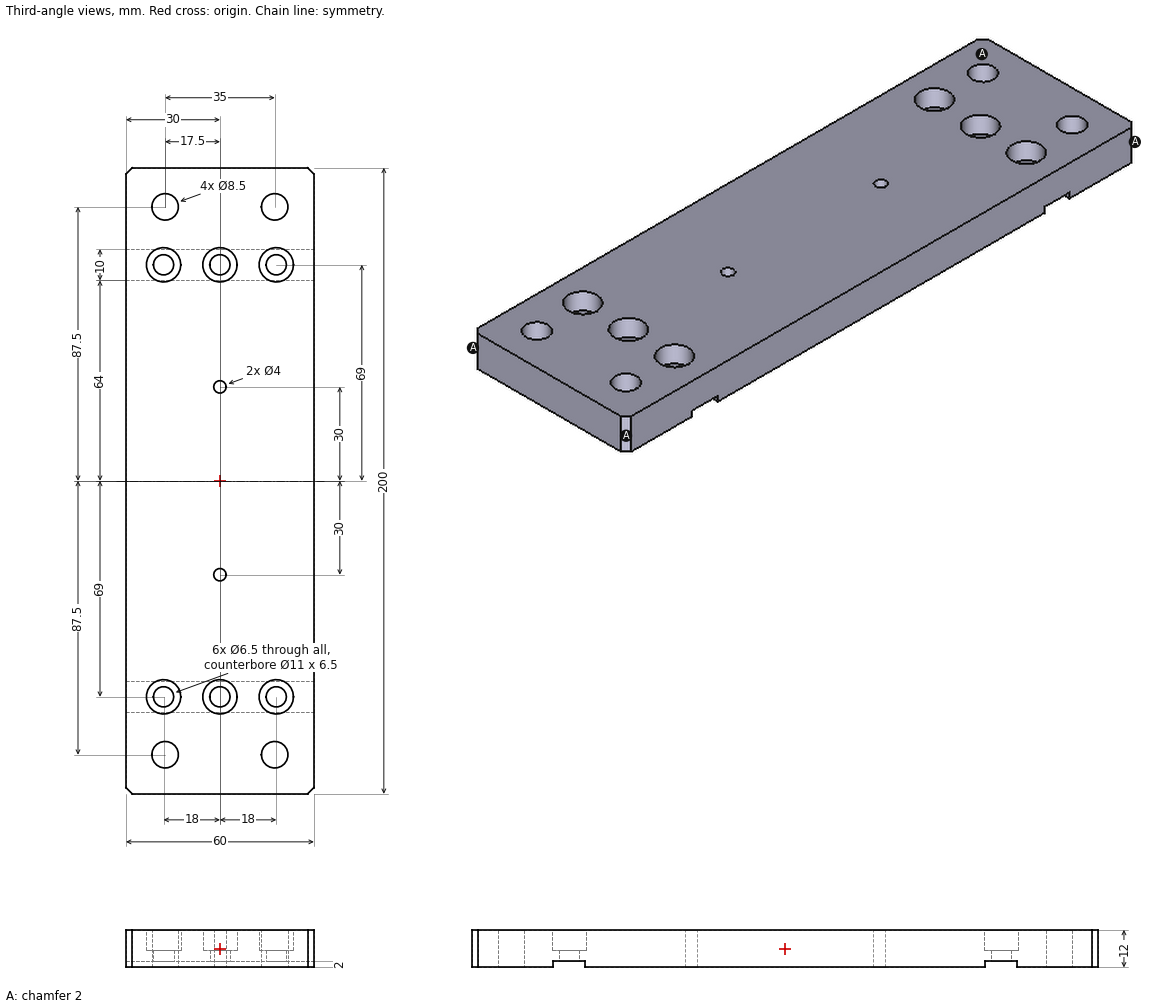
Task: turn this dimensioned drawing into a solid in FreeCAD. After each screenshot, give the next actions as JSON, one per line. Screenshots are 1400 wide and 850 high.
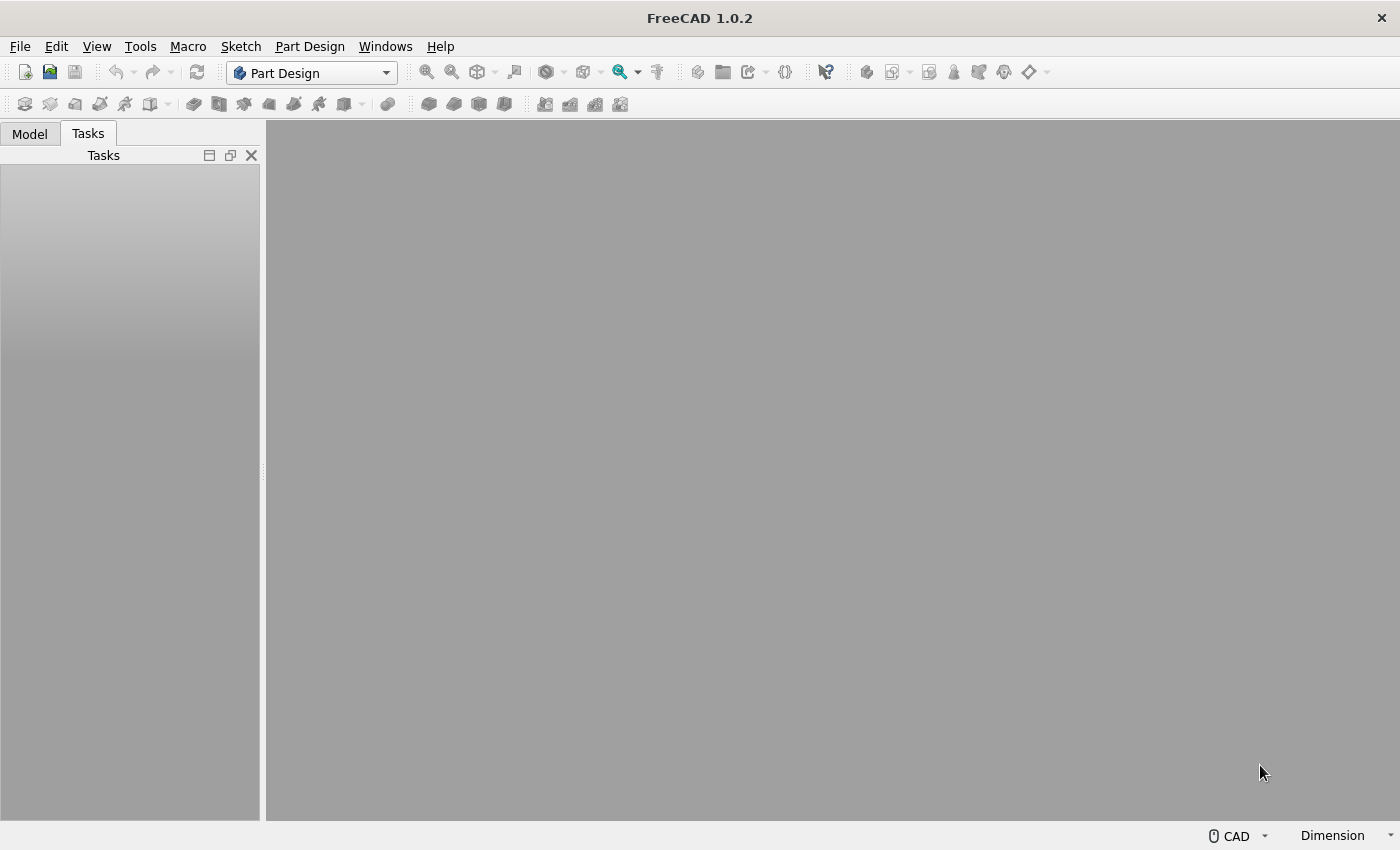
{"action": "left_click", "coordinate": [25, 72]}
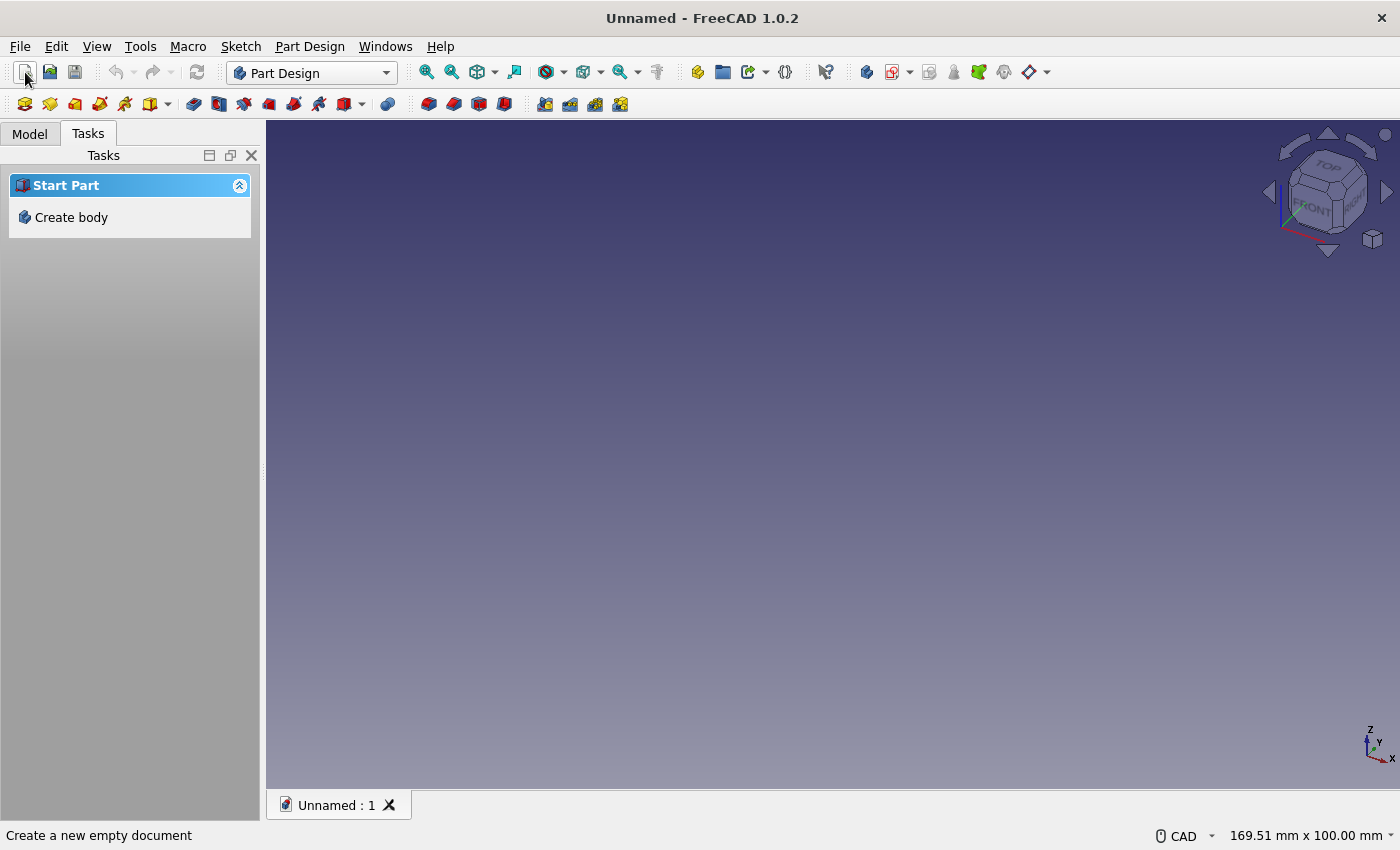
{"action": "left_click", "coordinate": [892, 72]}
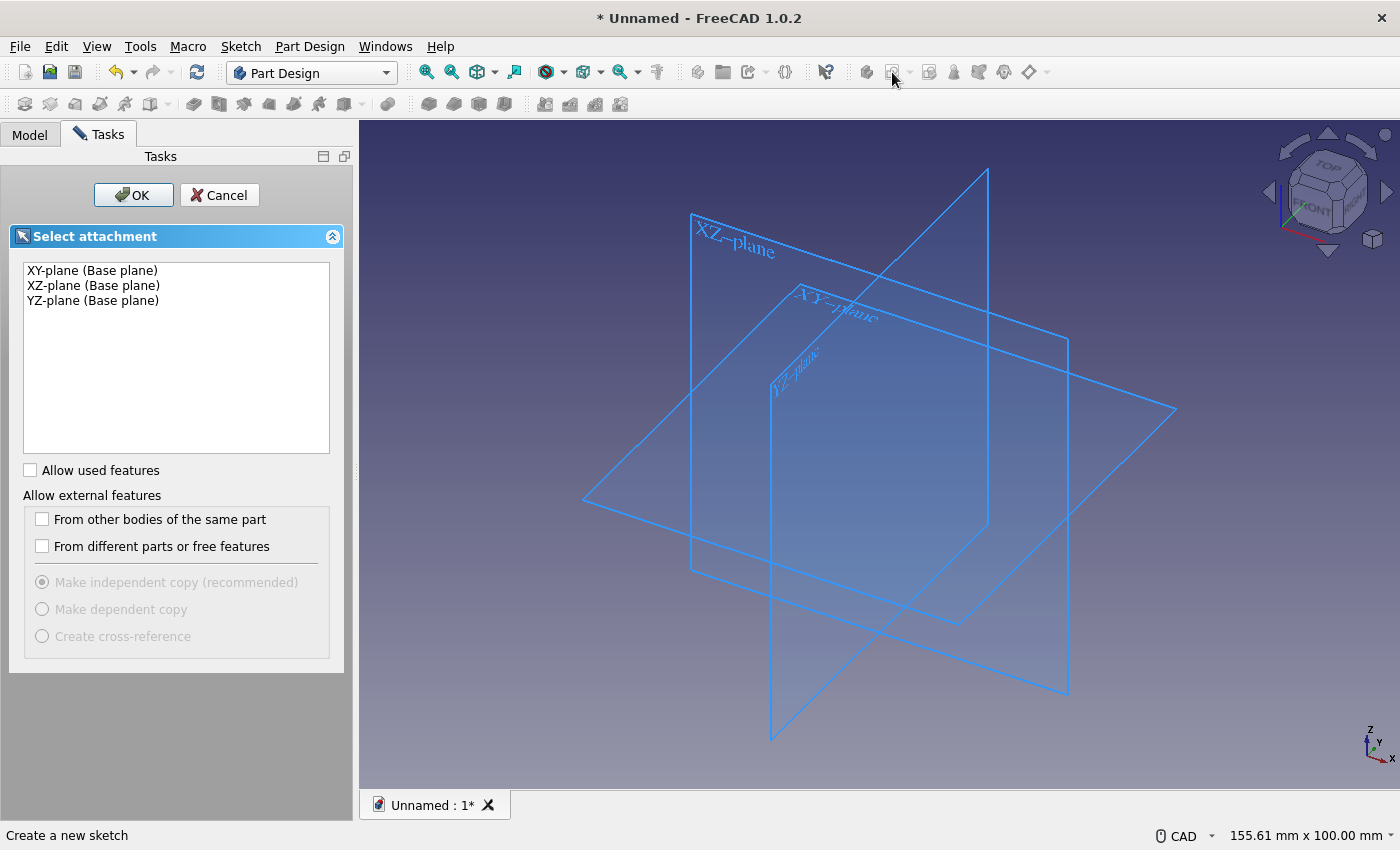
{"action": "left_click", "coordinate": [84, 270]}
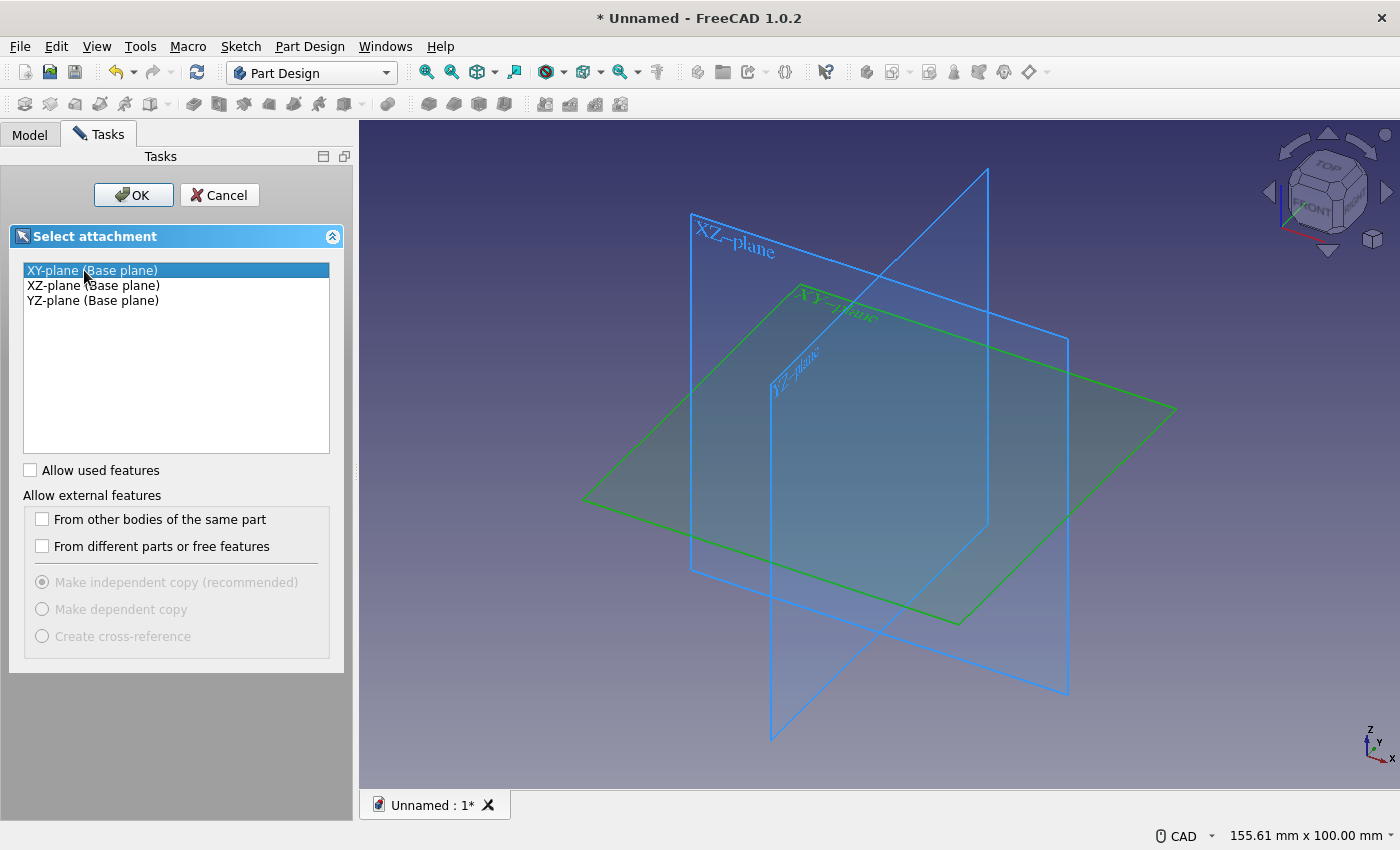
{"action": "left_click", "coordinate": [134, 195]}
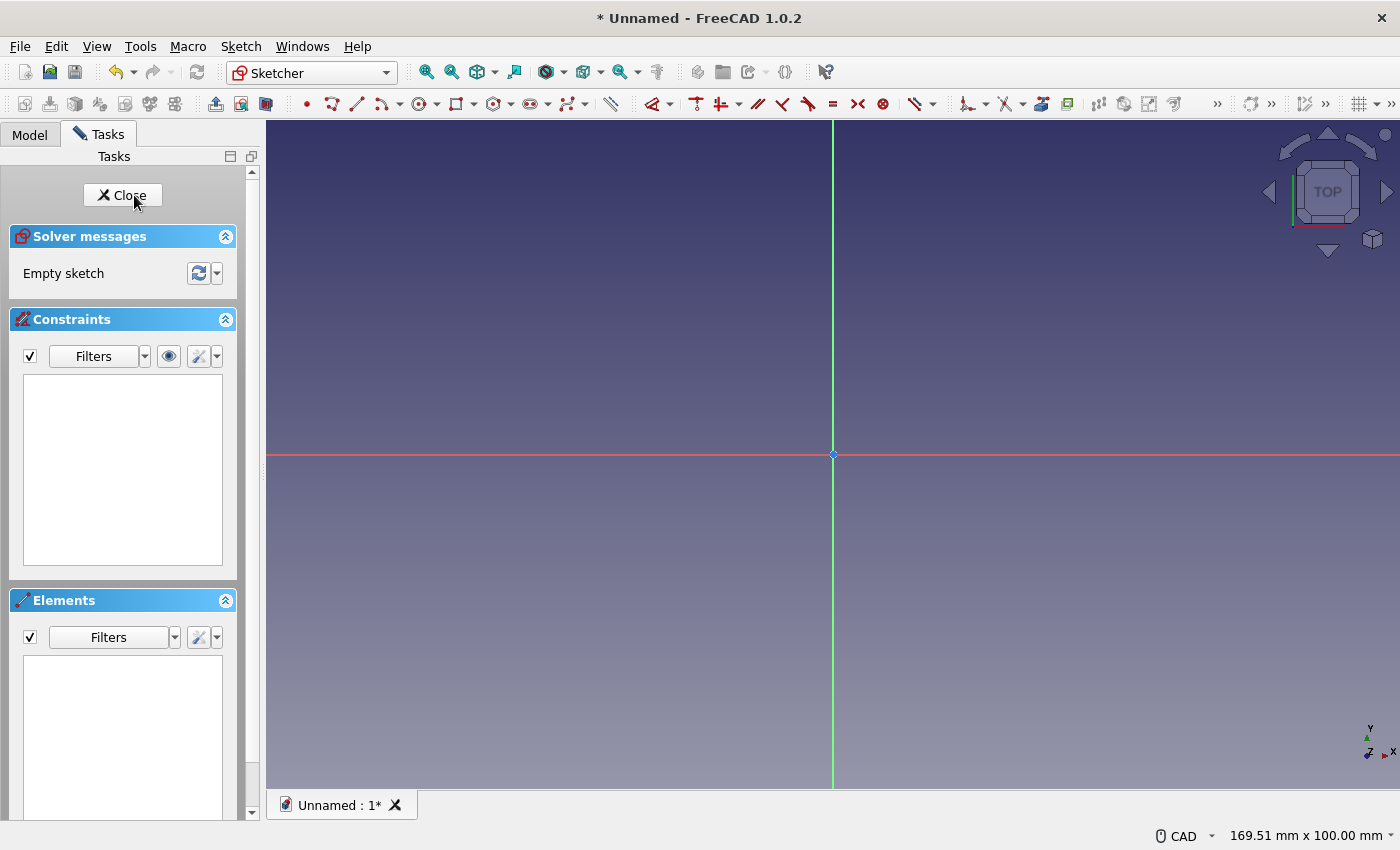
{"action": "scroll", "coordinate": [735, 454], "scroll_direction": "down", "scroll_amount": 6}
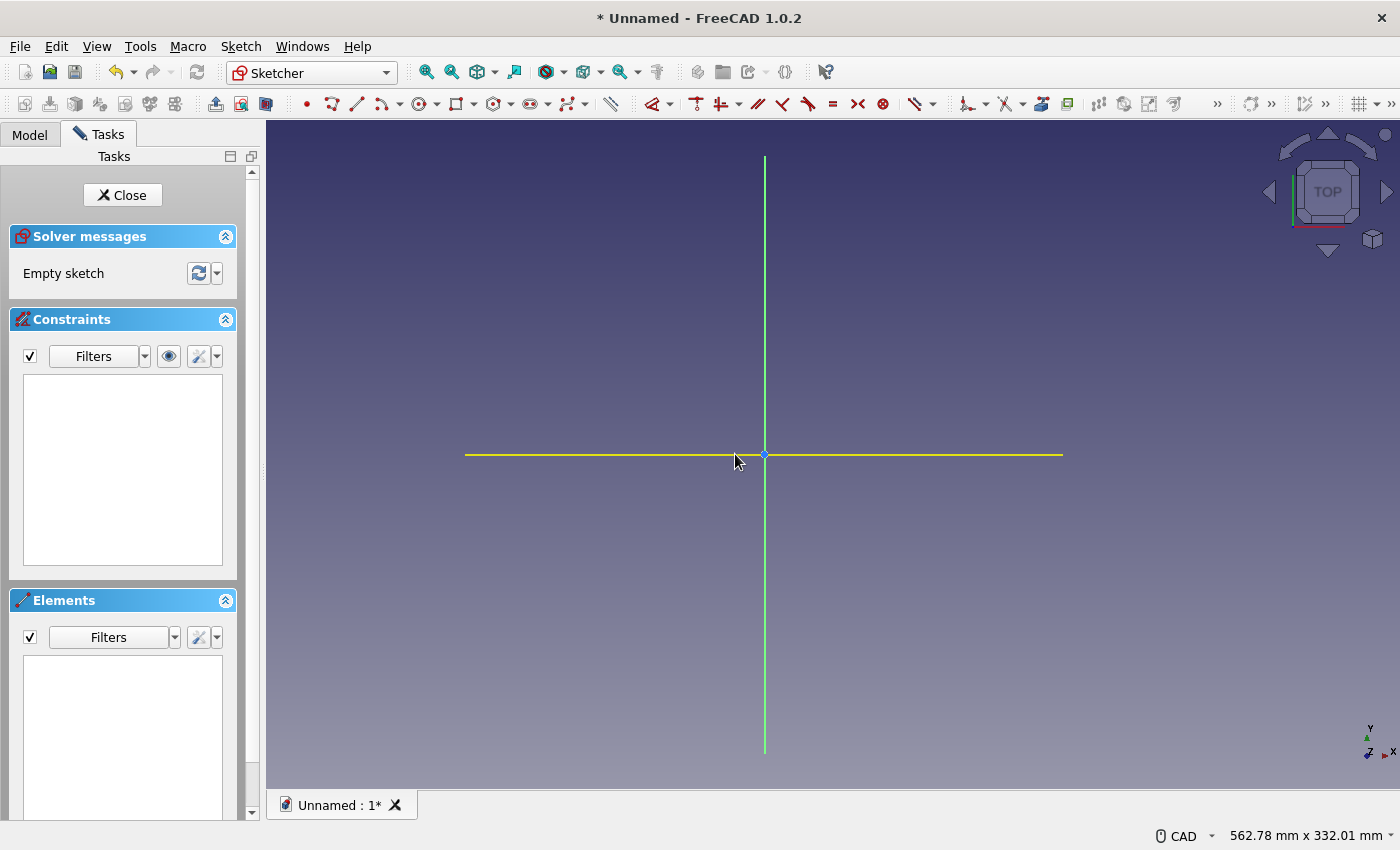
{"action": "left_click", "coordinate": [474, 104]}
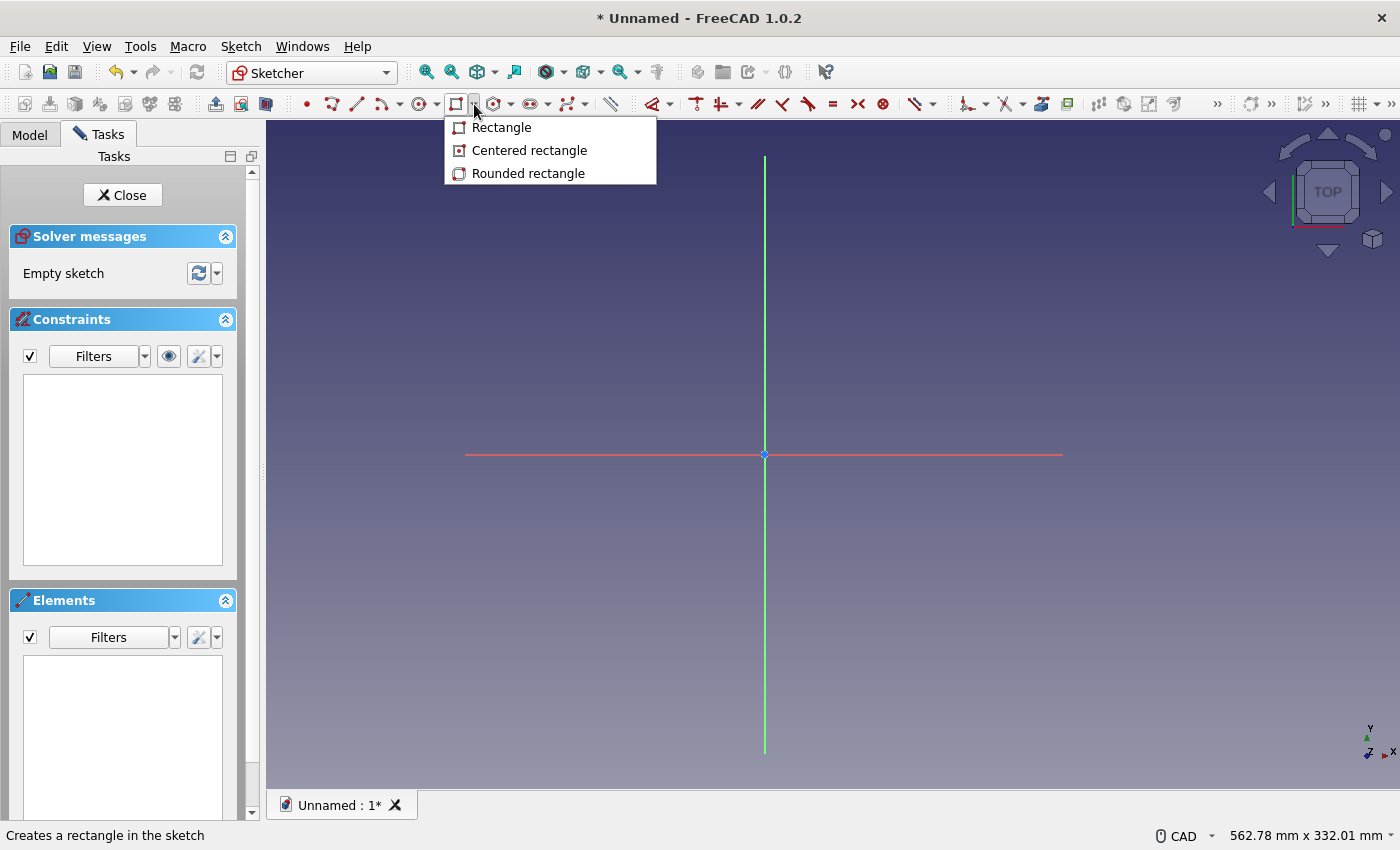
{"action": "left_click", "coordinate": [550, 150]}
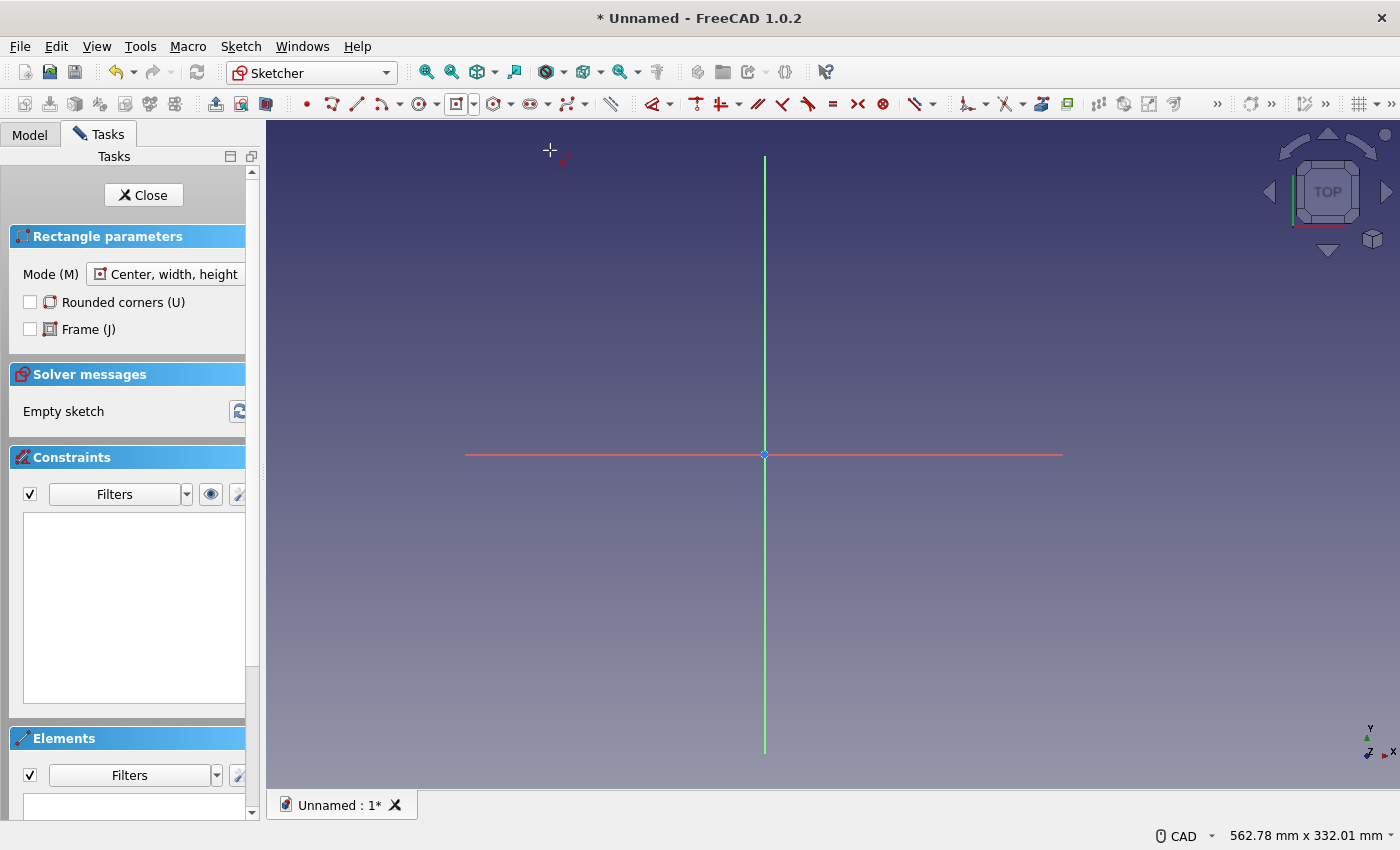
{"action": "left_click", "coordinate": [765, 454]}
{"action": "left_click", "coordinate": [825, 253]}
{"action": "key", "text": "Escape"}